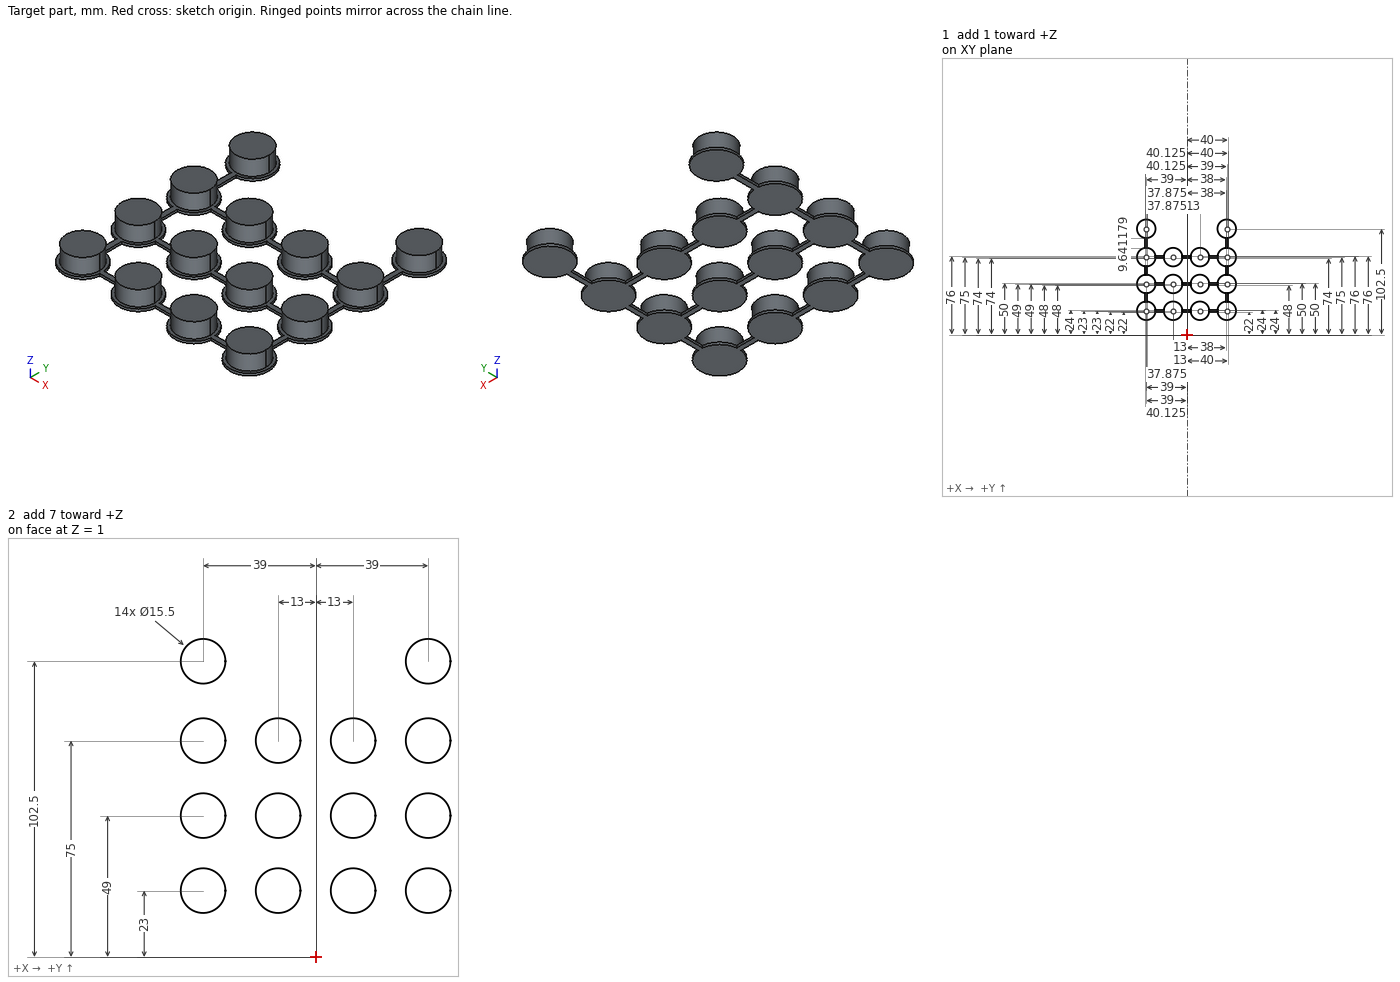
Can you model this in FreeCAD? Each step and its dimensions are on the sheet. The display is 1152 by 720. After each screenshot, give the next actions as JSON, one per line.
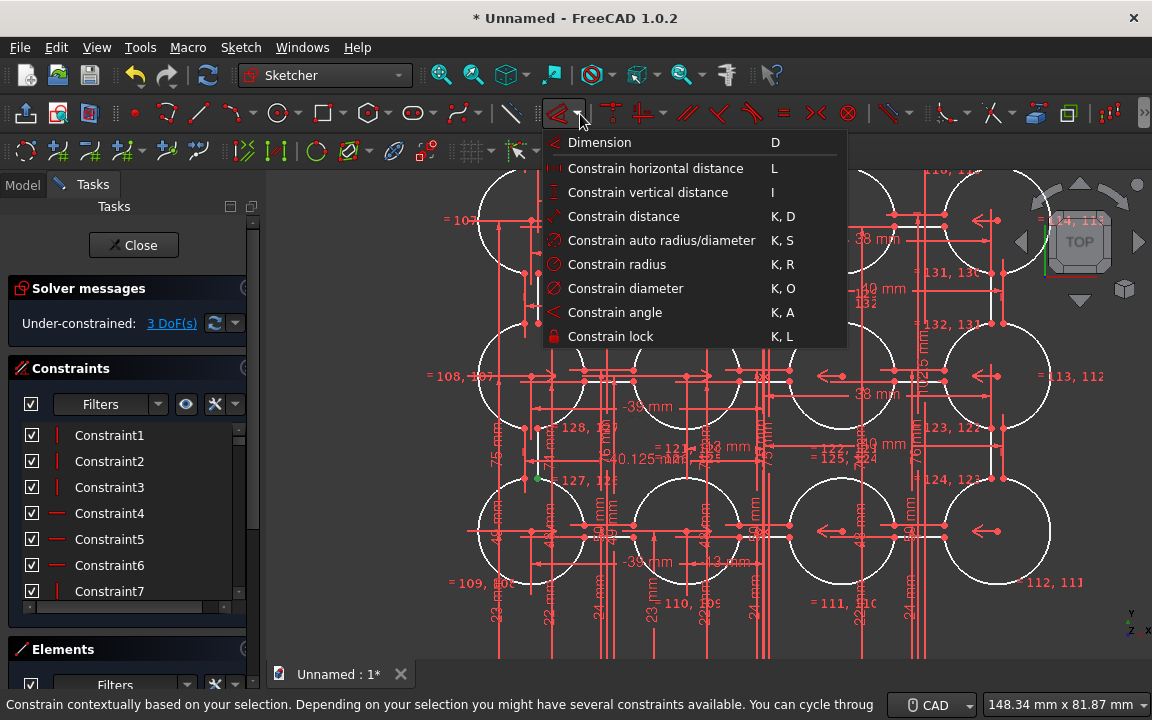
{"action": "left_click", "coordinate": [695, 168]}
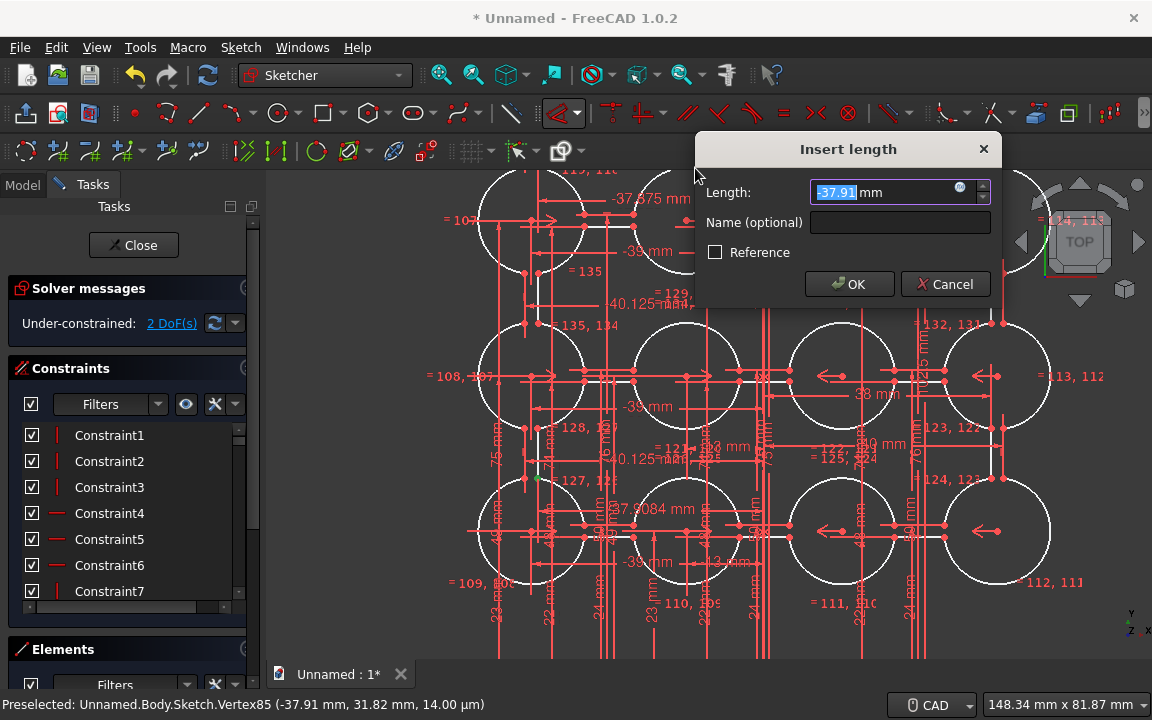
{"action": "type", "text": "-37.875"}
{"action": "key", "text": "Return"}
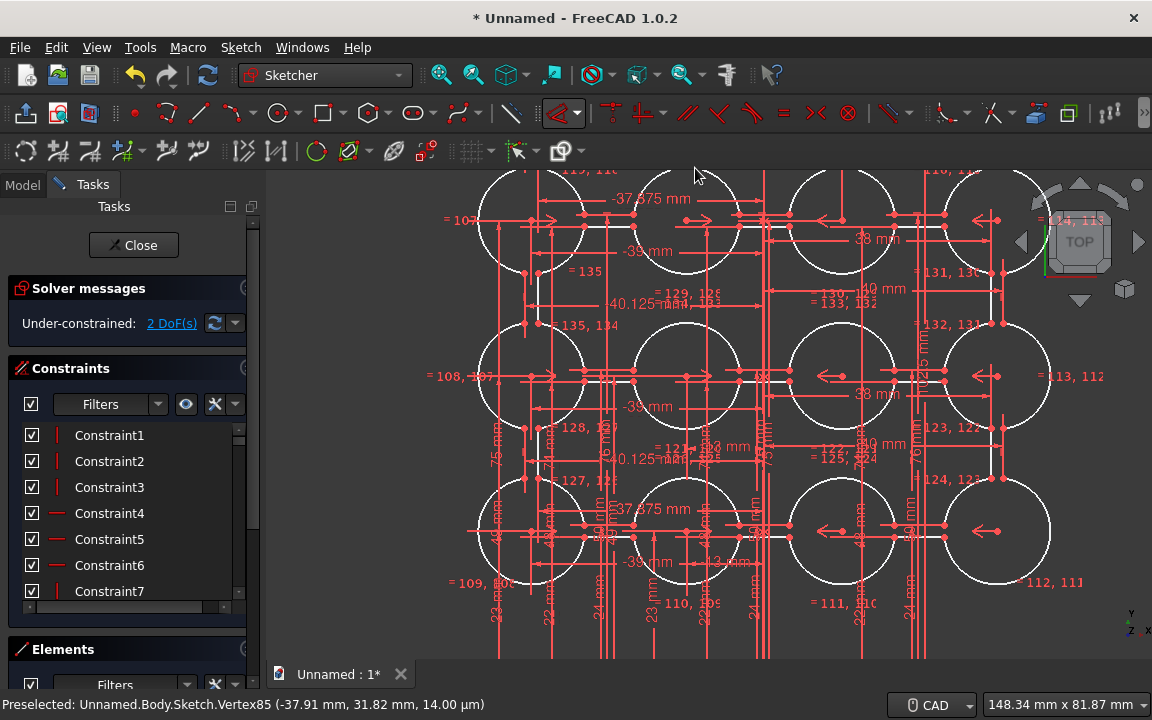
{"action": "left_click", "coordinate": [538, 323]}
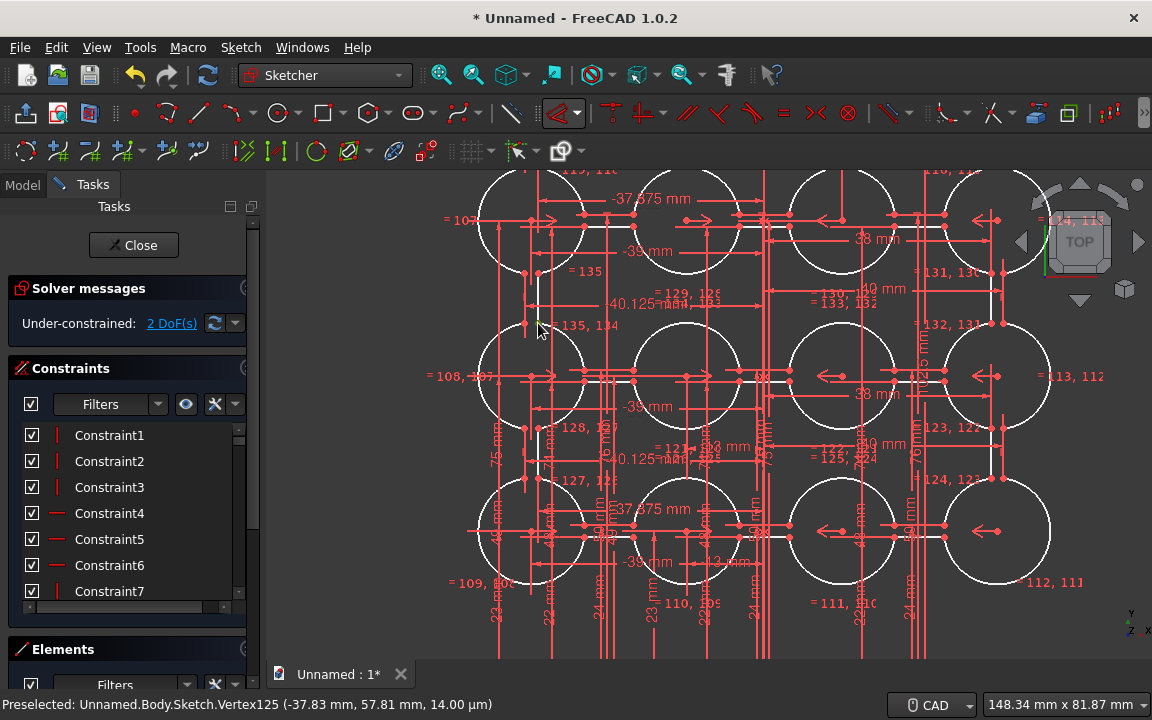
{"action": "left_click", "coordinate": [580, 114]}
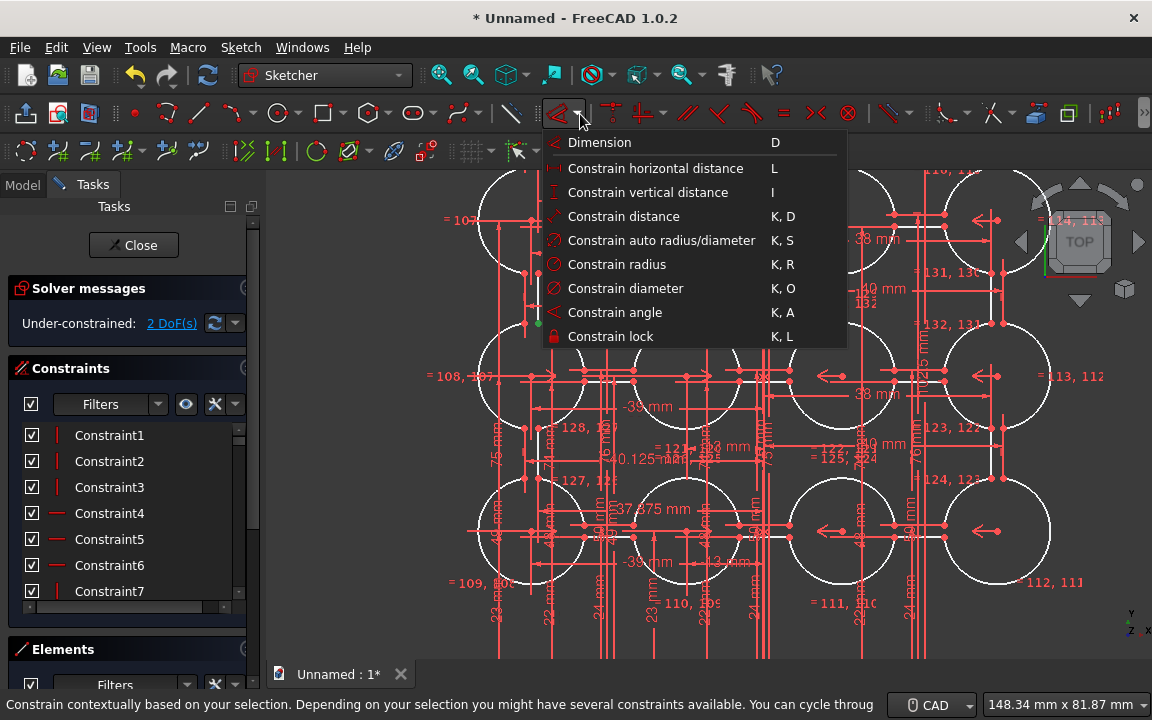
{"action": "left_click", "coordinate": [695, 168]}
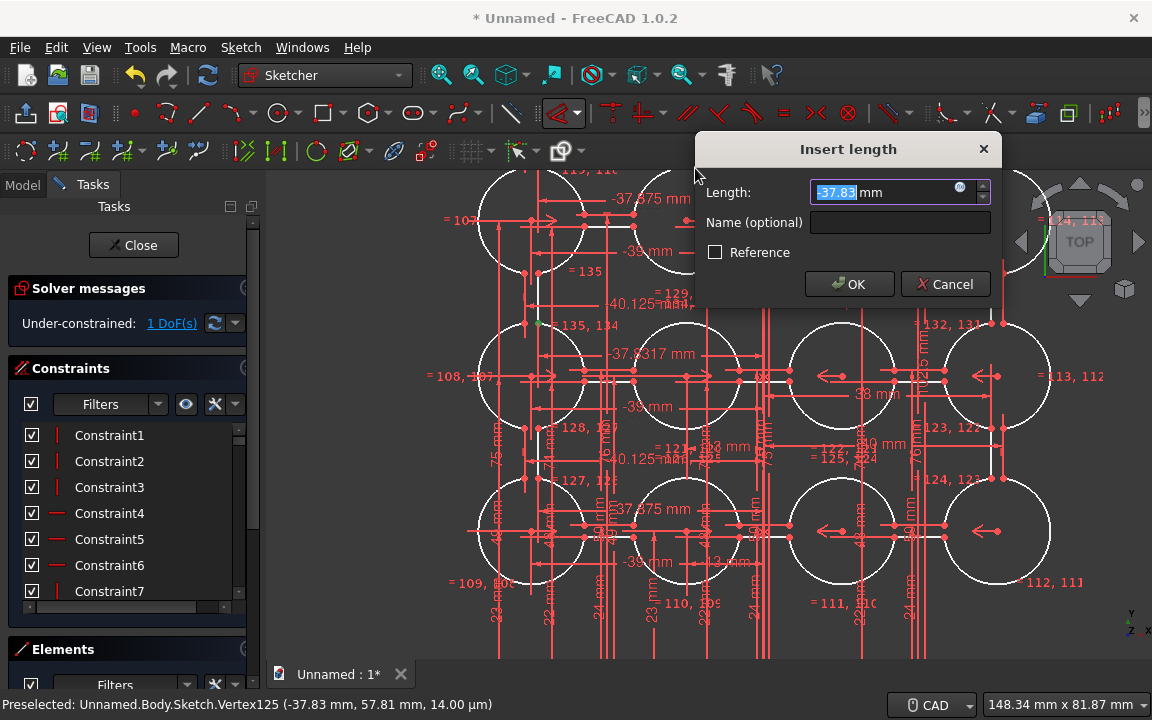
{"action": "type", "text": "-37.875"}
{"action": "key", "text": "Return"}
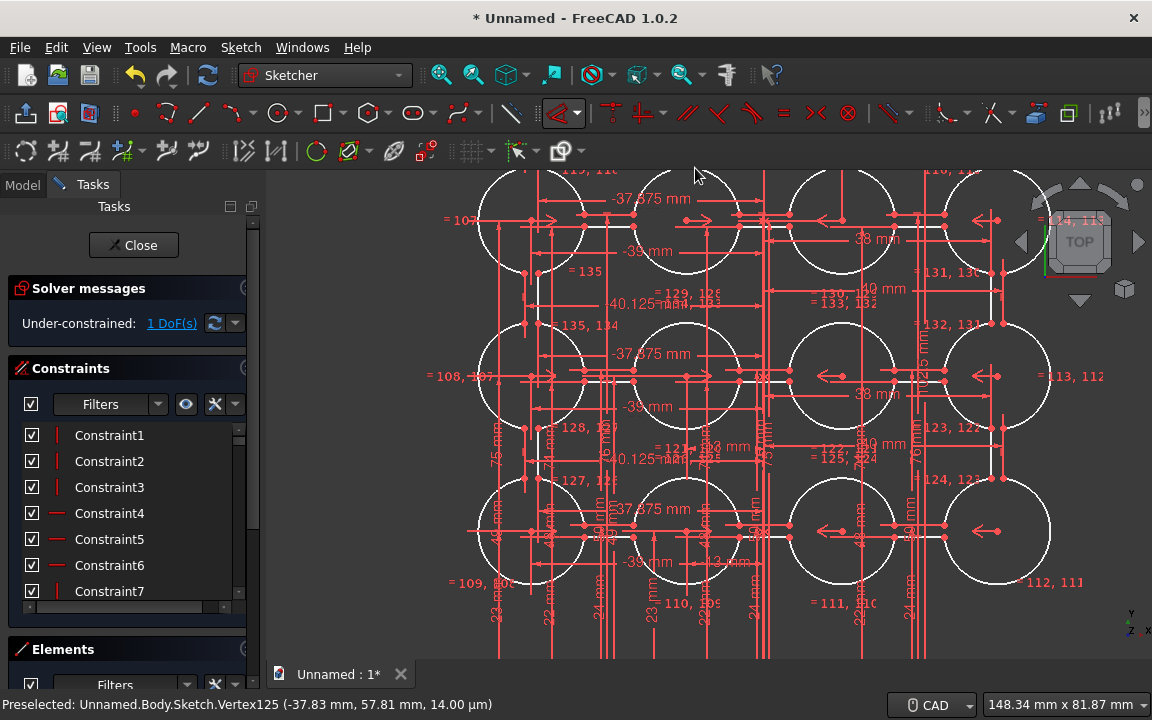
{"action": "scroll", "coordinate": [539, 479], "scroll_direction": "down", "scroll_amount": 4}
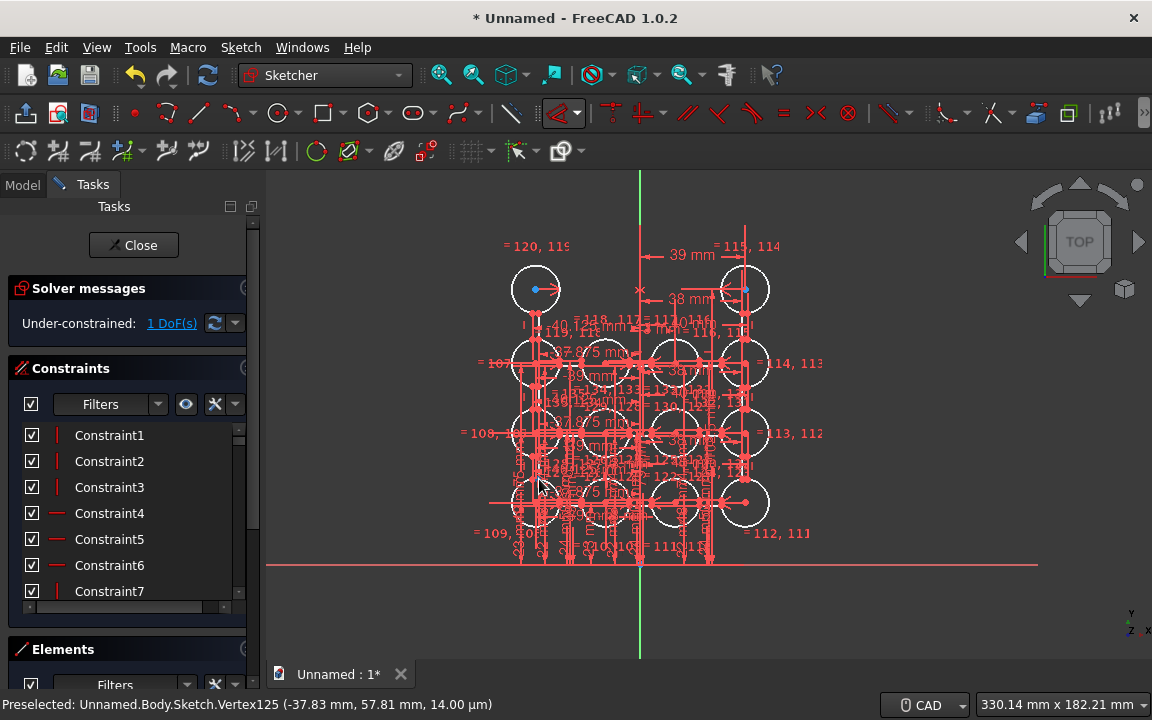
{"action": "scroll", "coordinate": [533, 321], "scroll_direction": "up", "scroll_amount": 5}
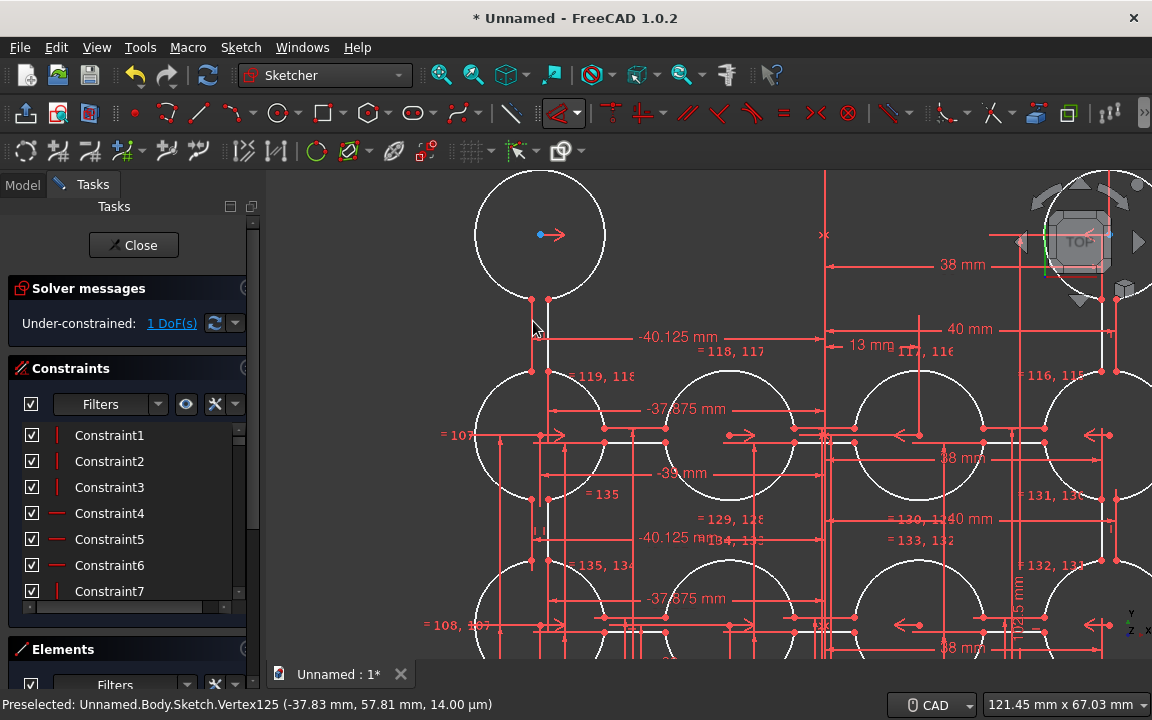
{"action": "left_click", "coordinate": [532, 321]}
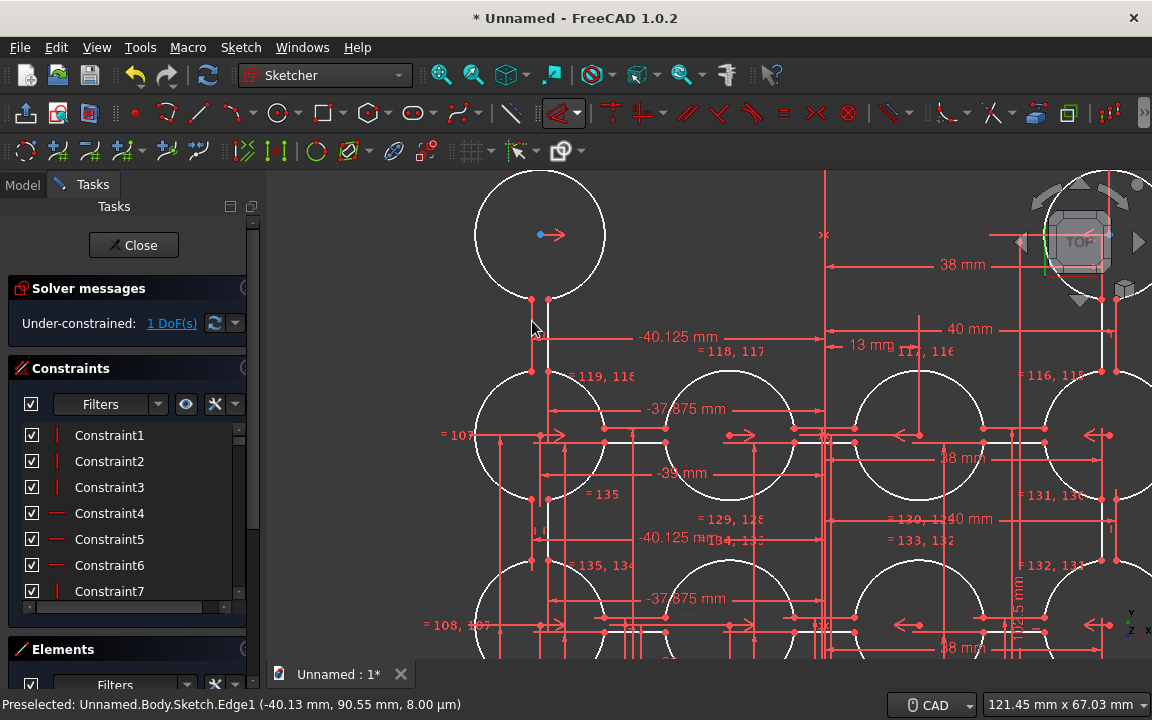
{"action": "left_click", "coordinate": [580, 114]}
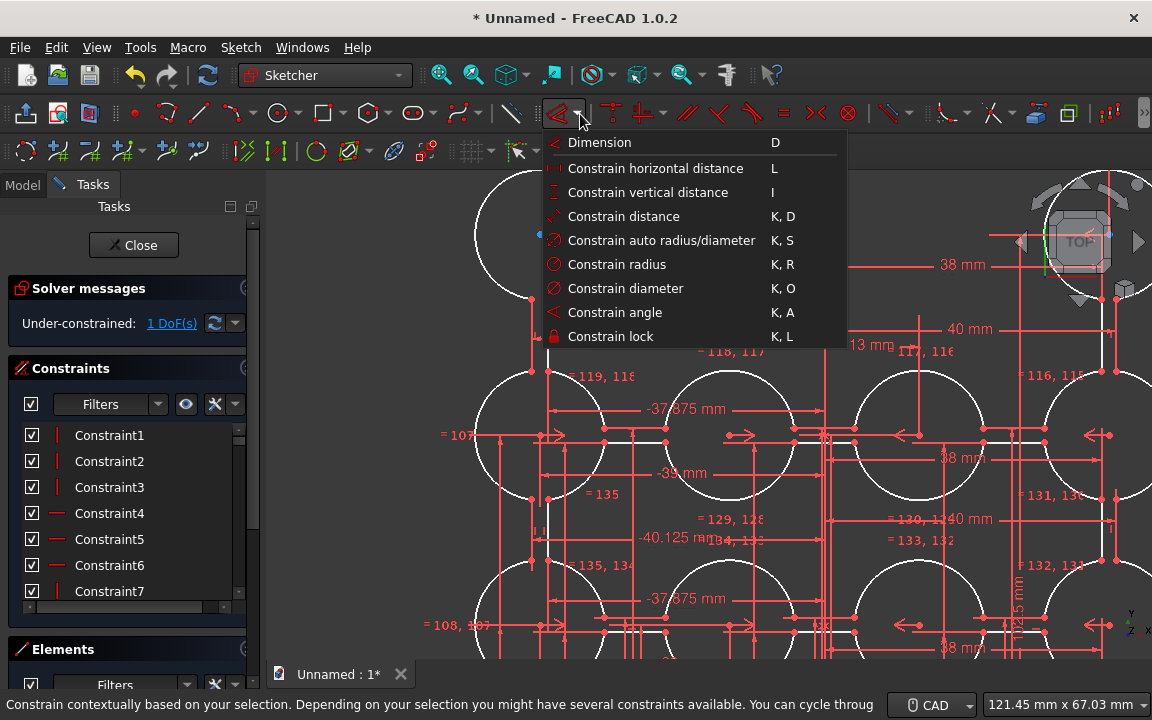
{"action": "left_click", "coordinate": [695, 192]}